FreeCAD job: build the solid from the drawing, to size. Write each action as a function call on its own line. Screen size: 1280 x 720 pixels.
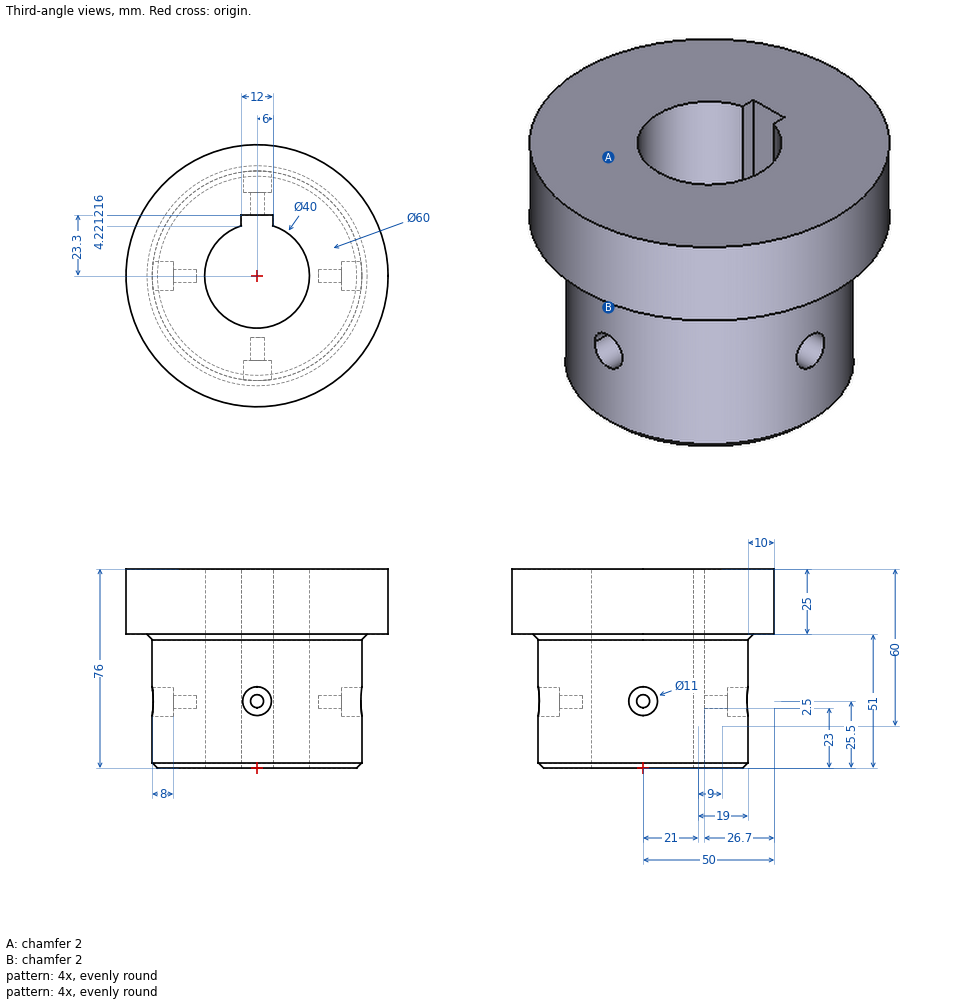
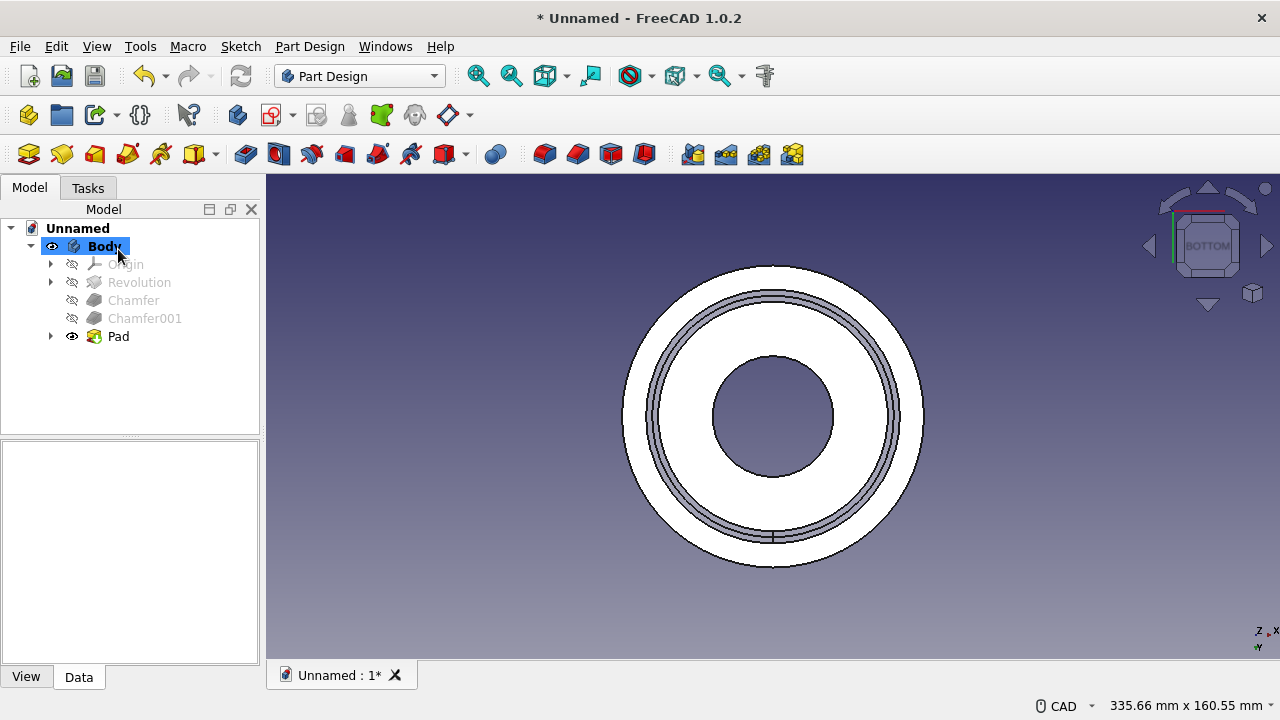
click(839, 350)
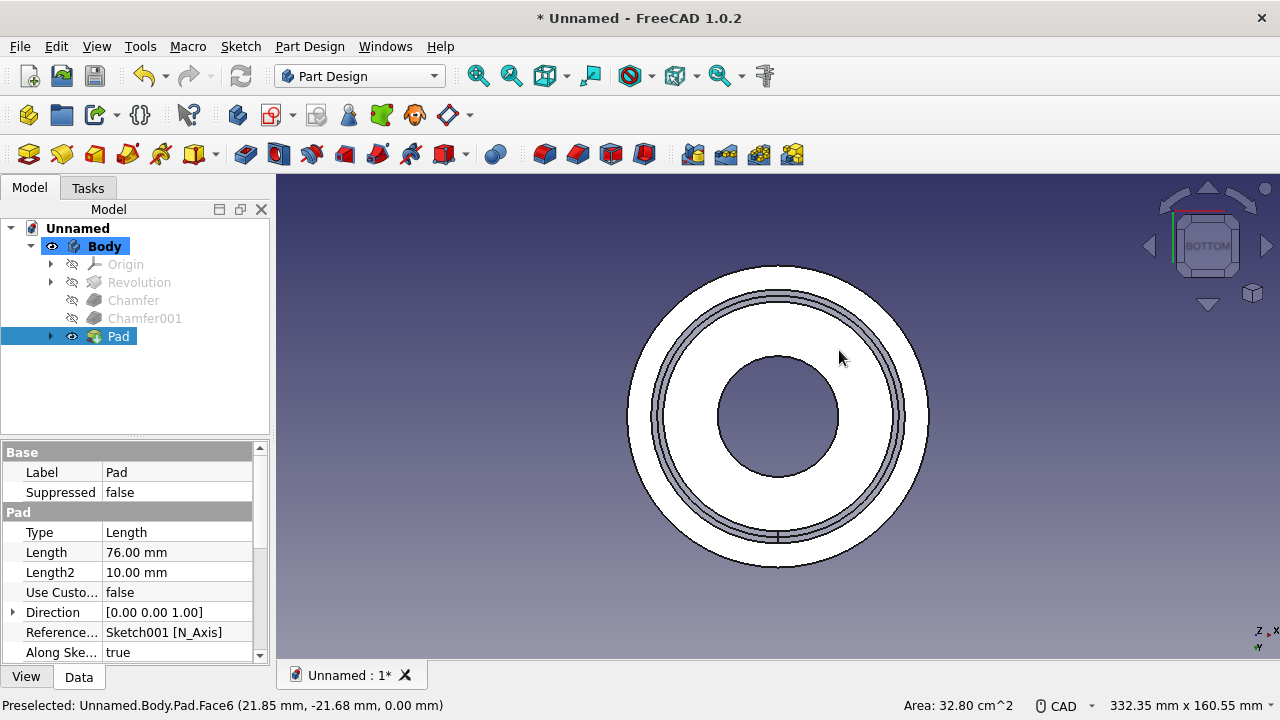
click(270, 116)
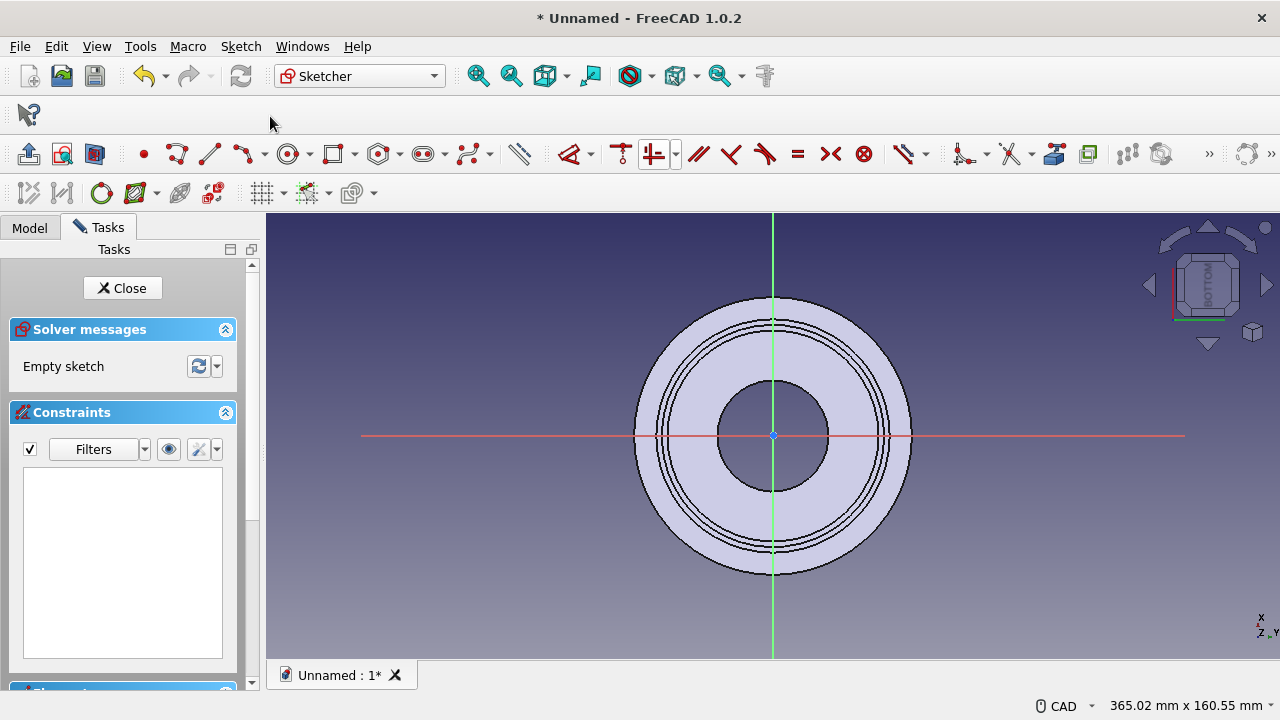
scroll(818, 436, up, 11)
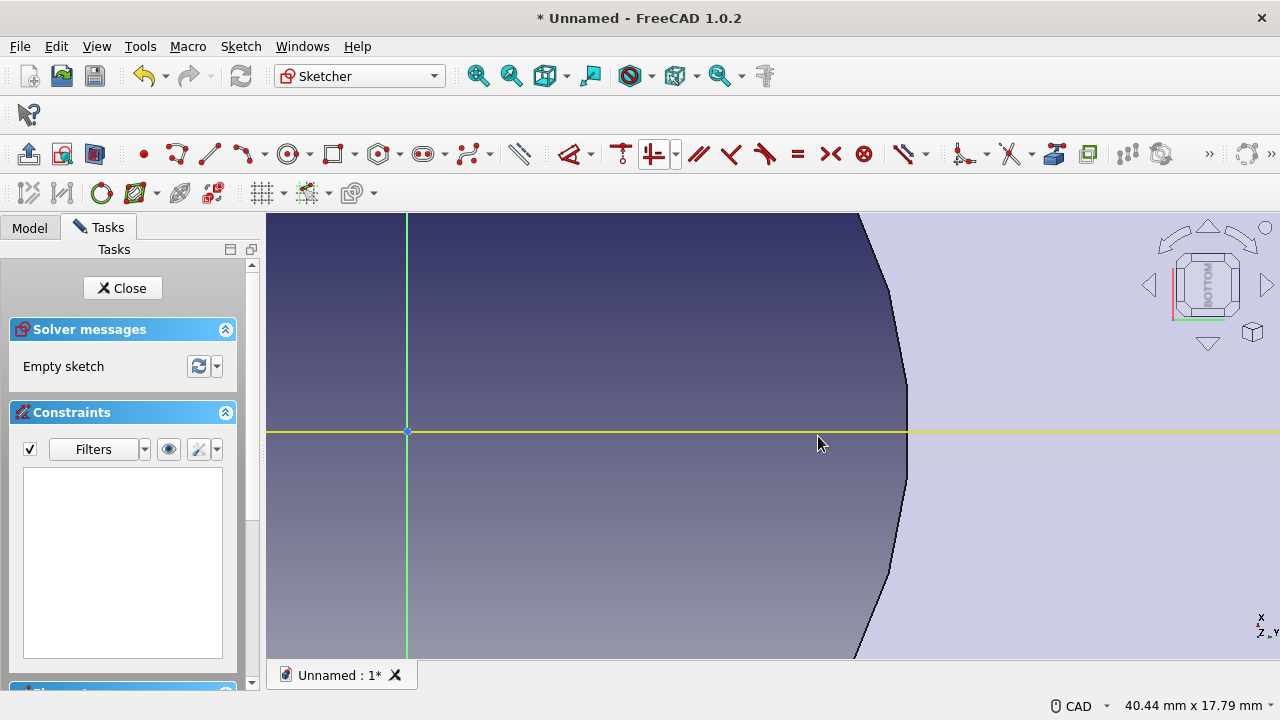
key(g)
key(r)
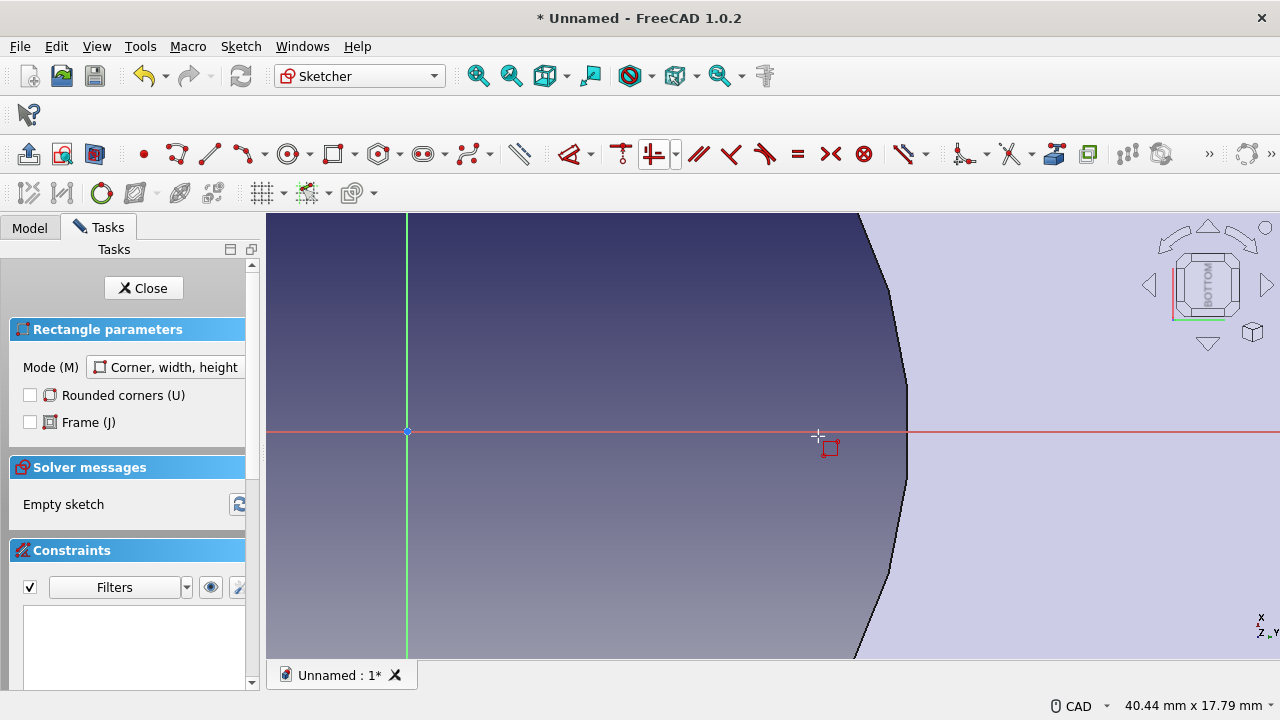
click(886, 282)
move(992, 582)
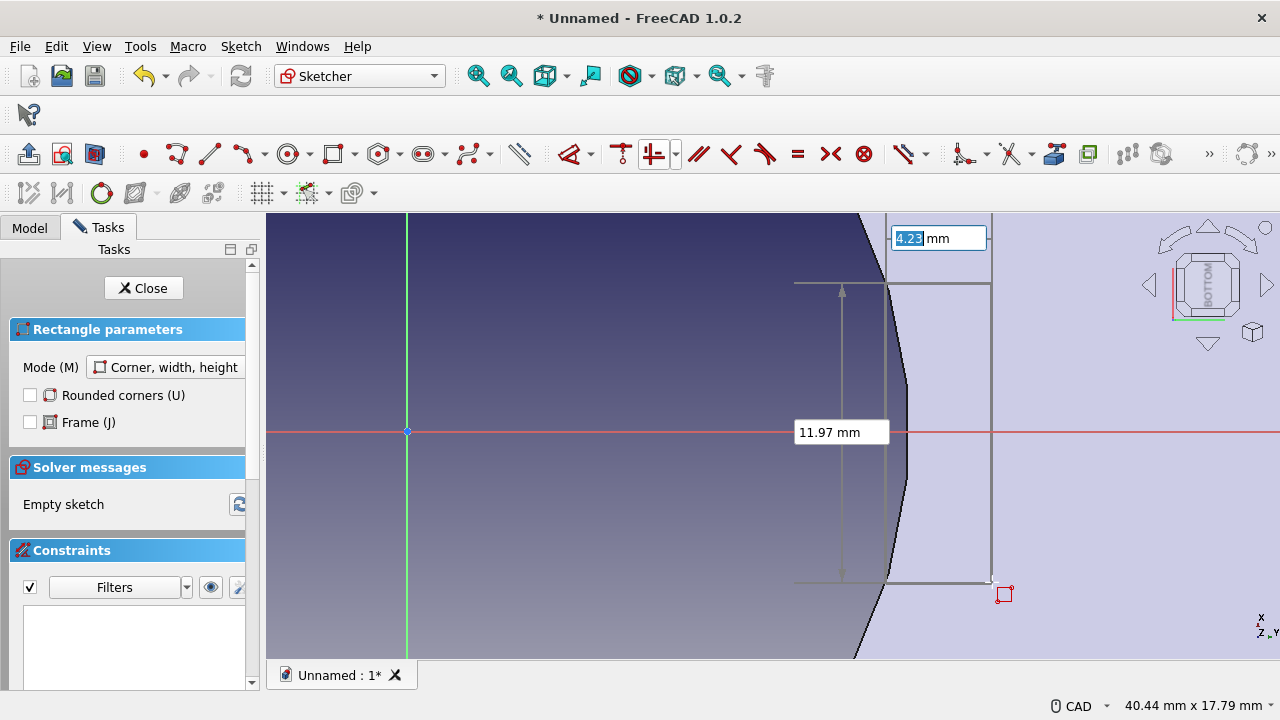
text(4.221216)
key(Tab)
text(12)
key(Return)
key(Escape)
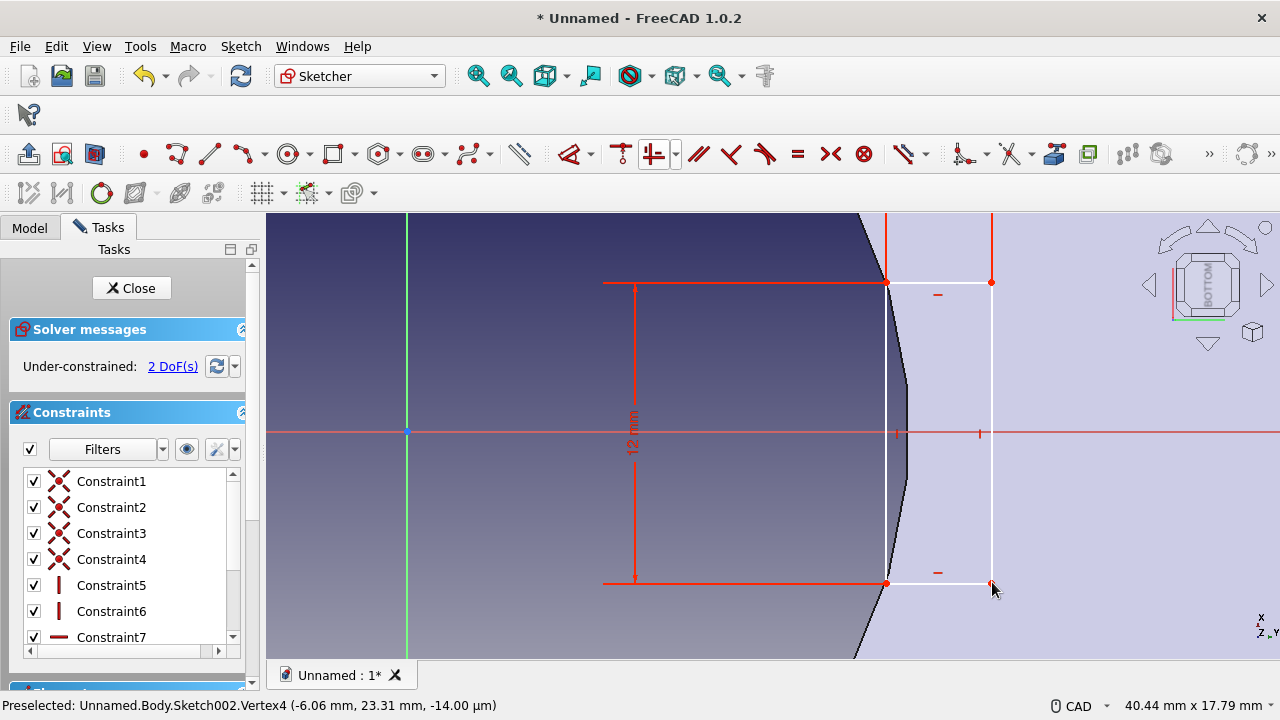
key(d)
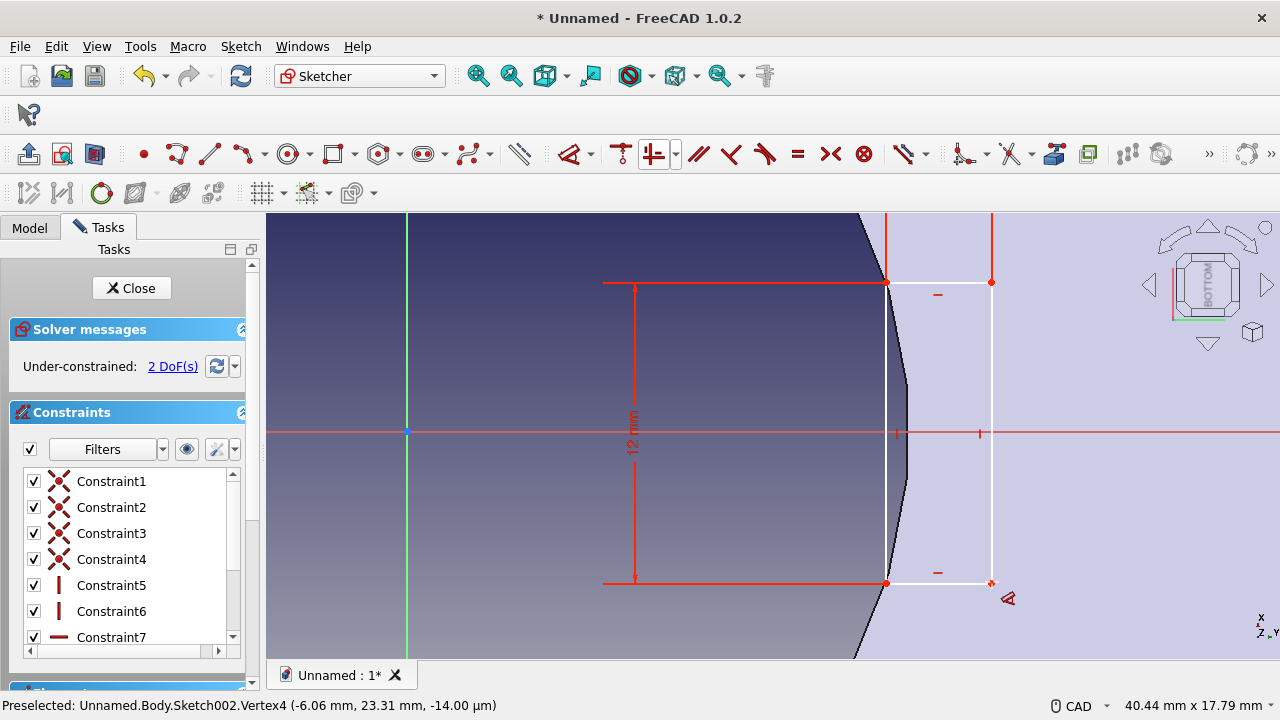
click(886, 283)
click(374, 357)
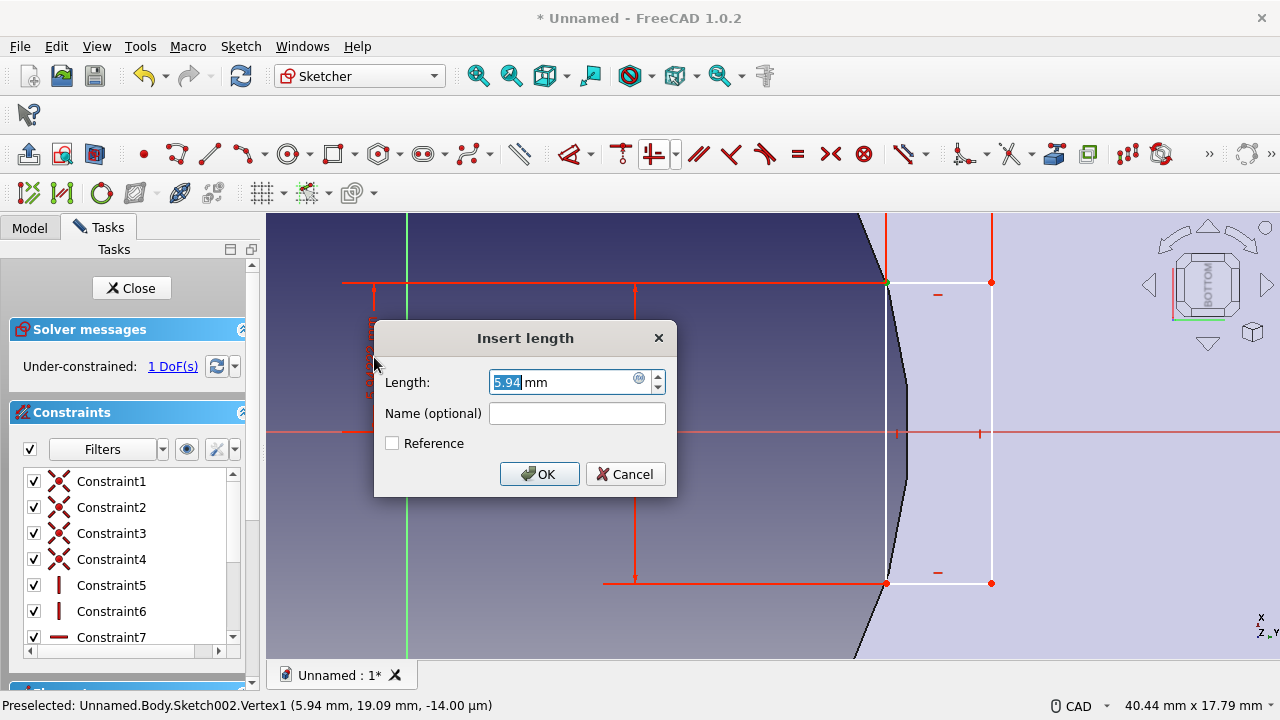
text(6)
key(Return)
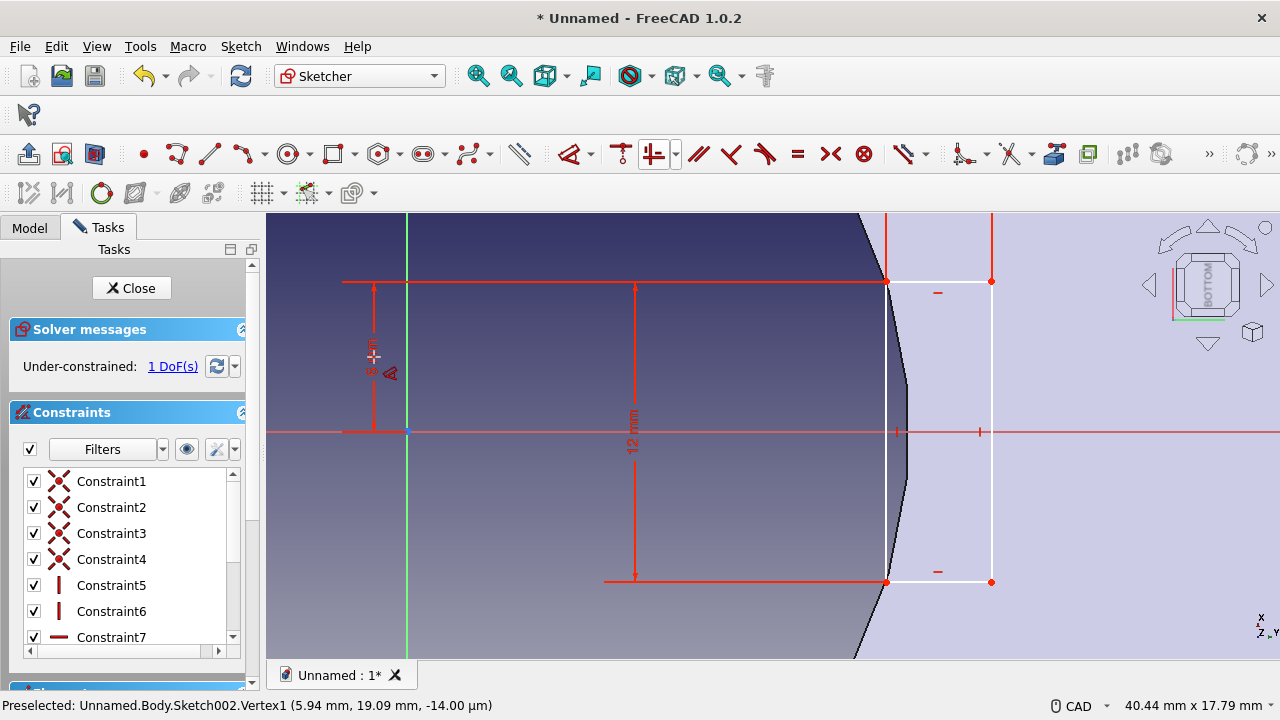
click(992, 582)
click(700, 616)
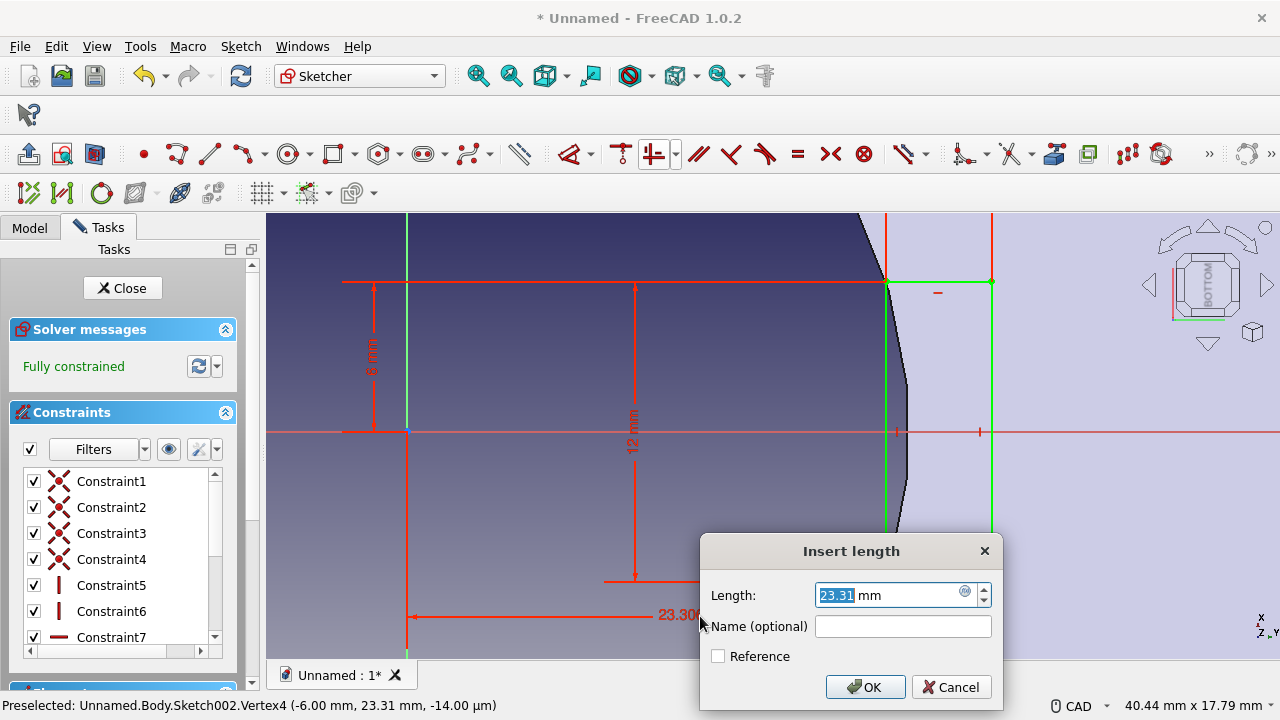
text(23.3)
key(Return)
key(Escape)